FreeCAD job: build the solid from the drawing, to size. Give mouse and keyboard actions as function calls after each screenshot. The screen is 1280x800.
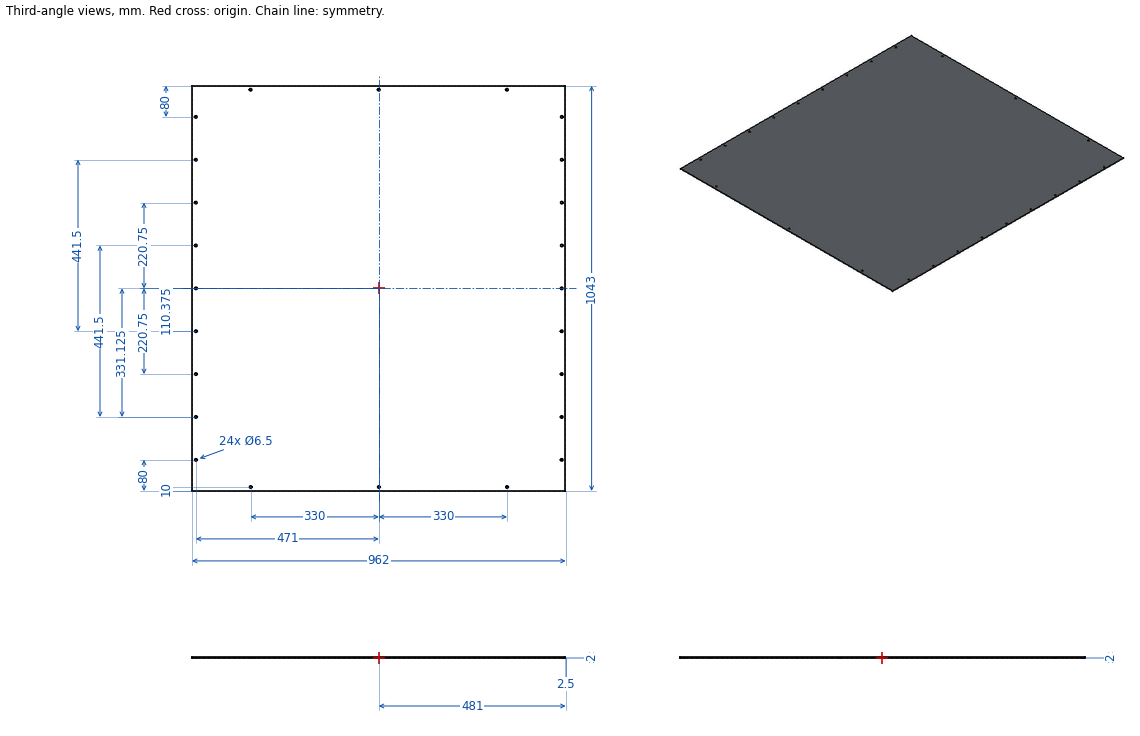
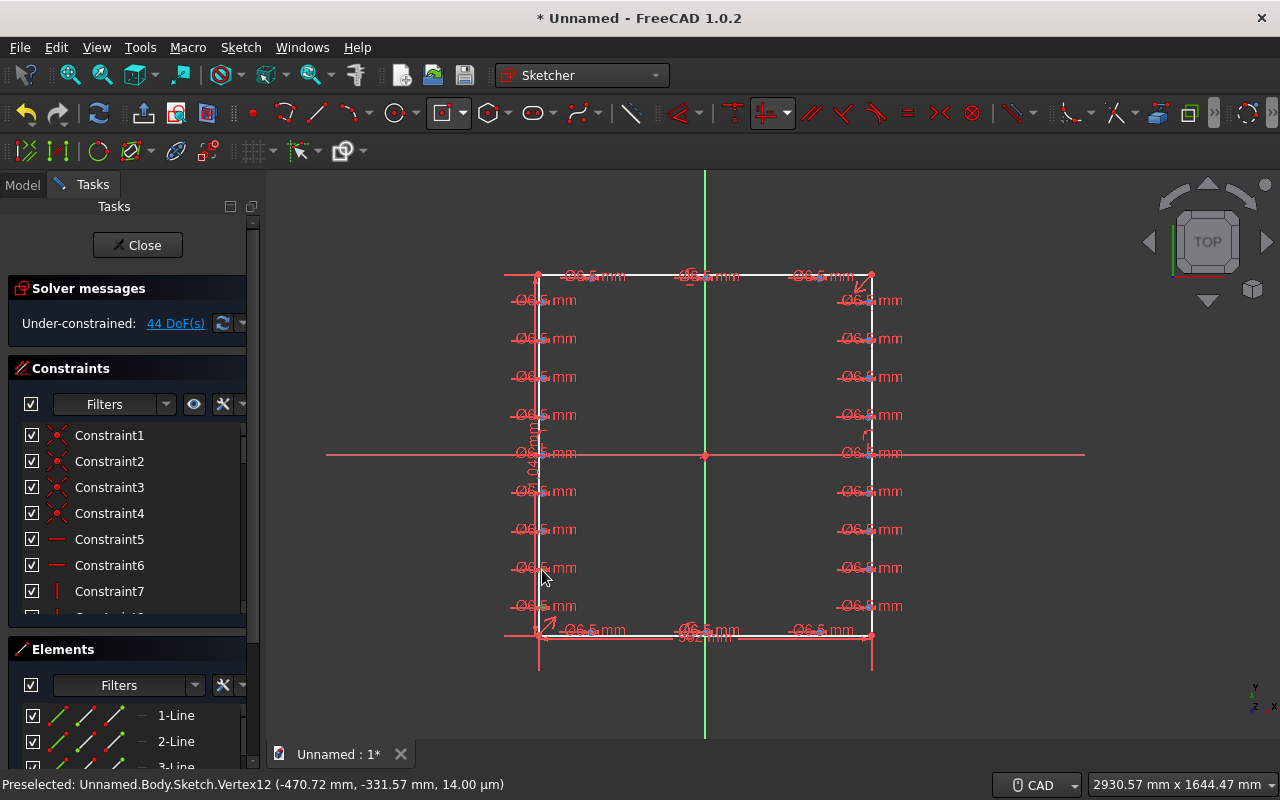
click(790, 114)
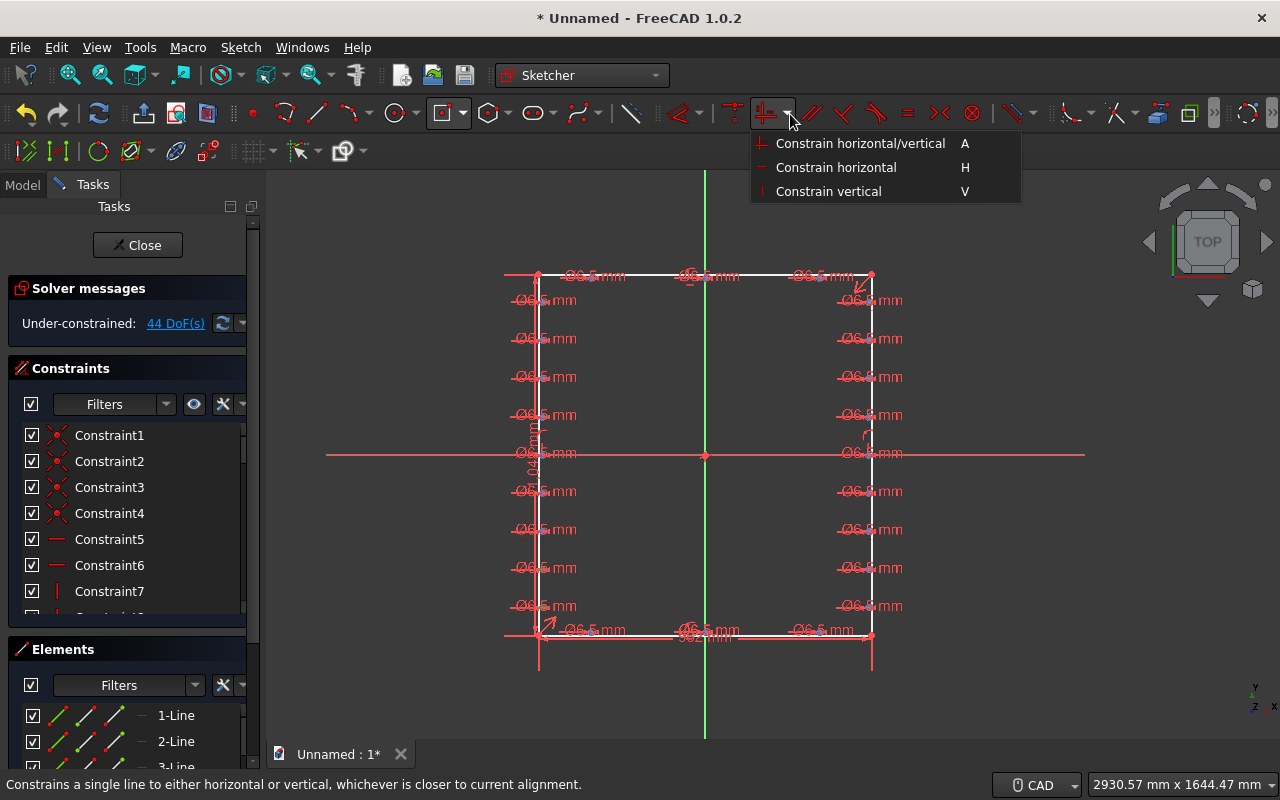
click(886, 191)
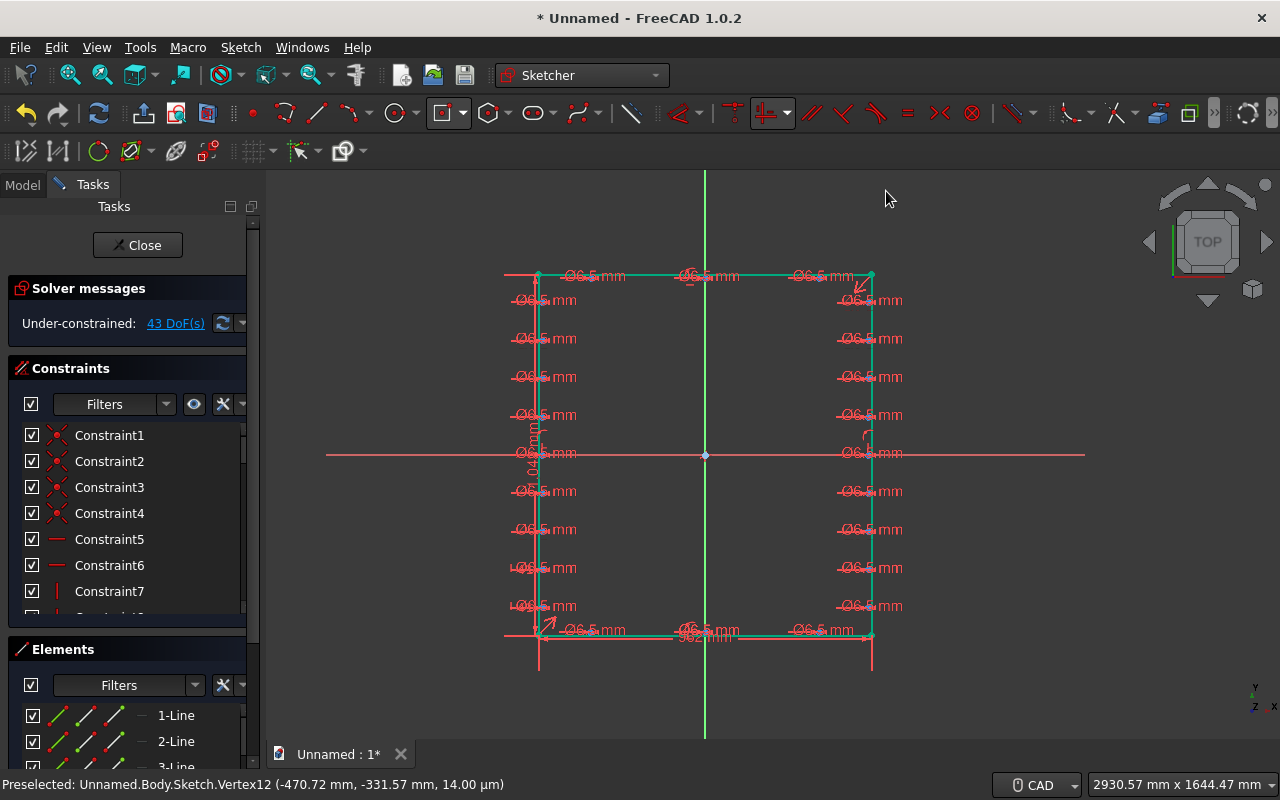
click(542, 570)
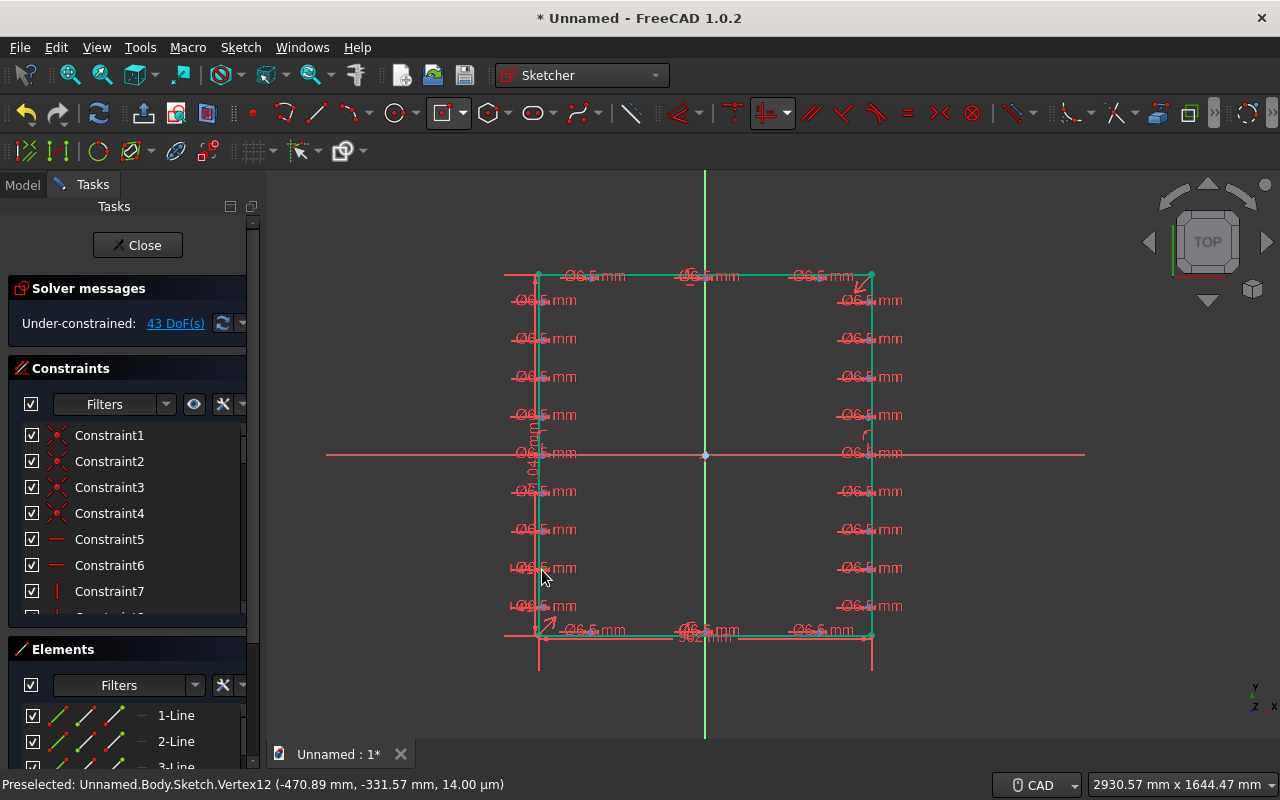
click(542, 532)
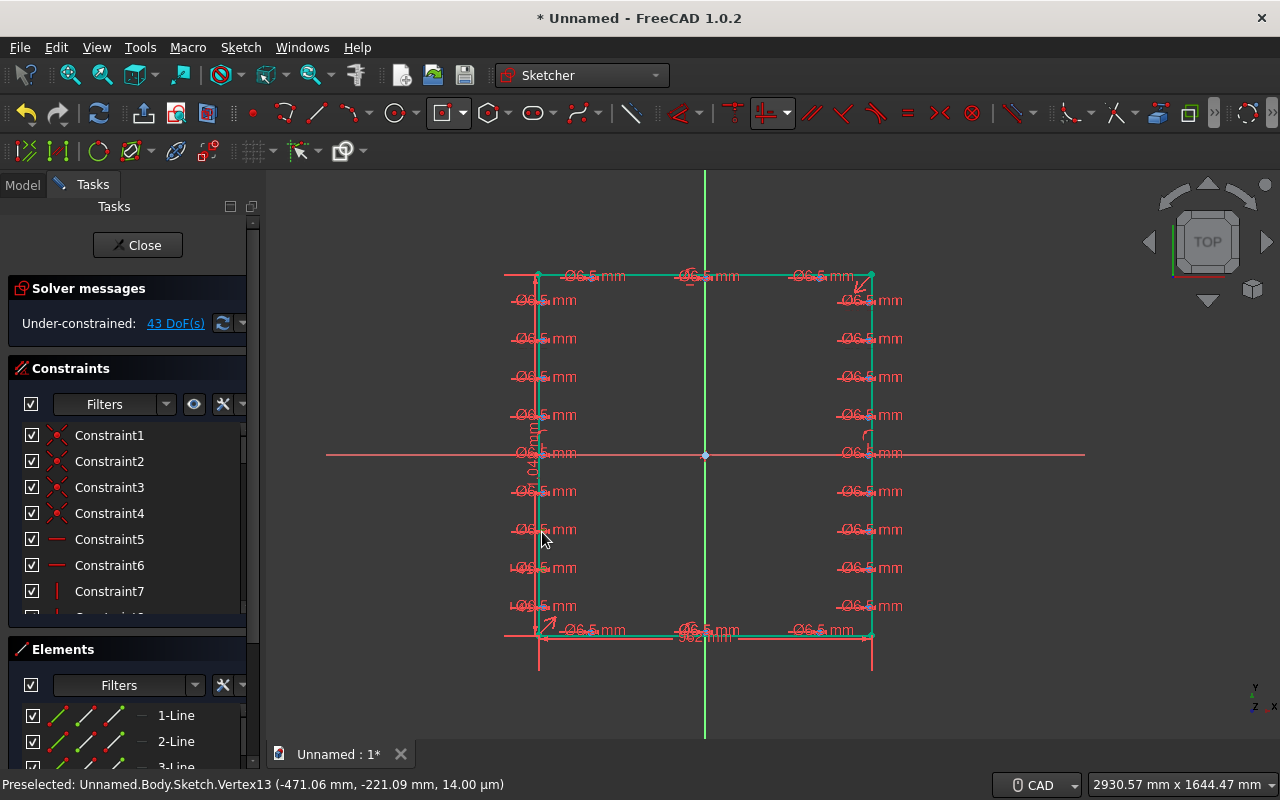
click(790, 114)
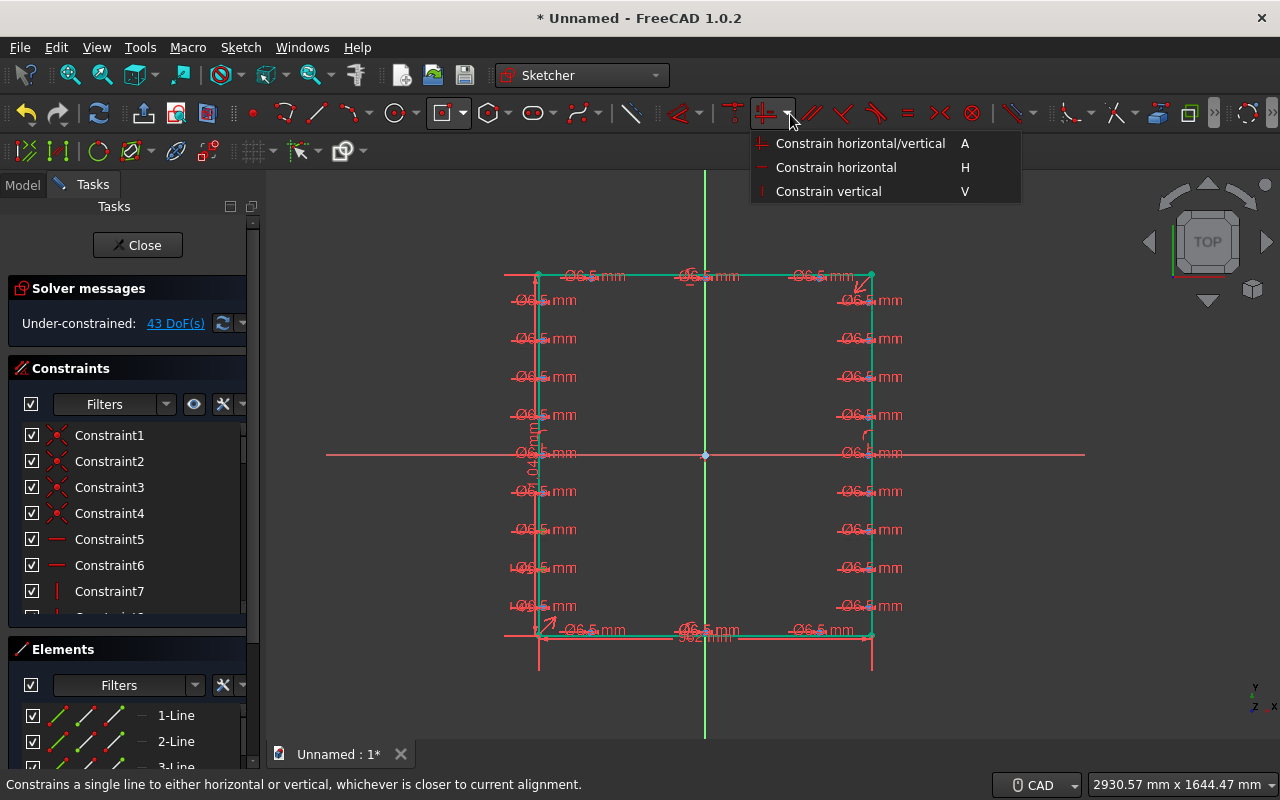
click(886, 191)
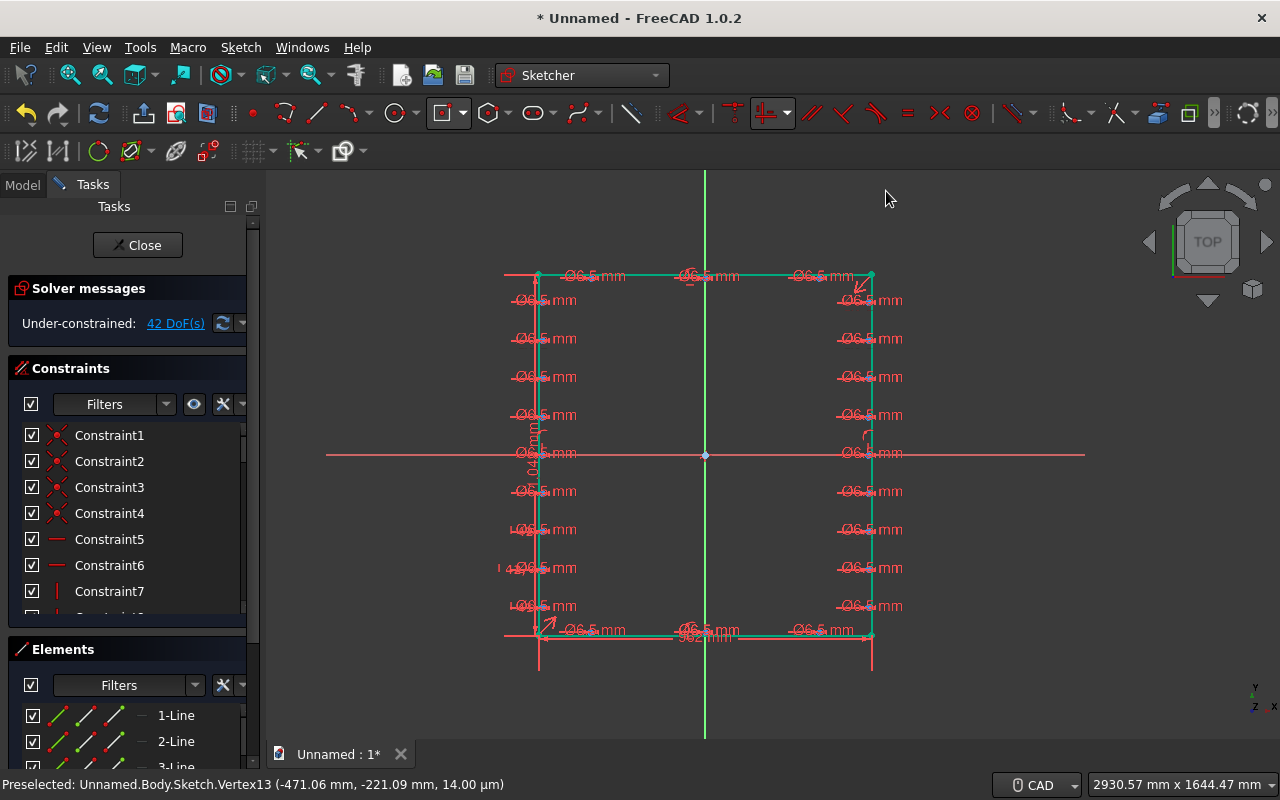
click(542, 532)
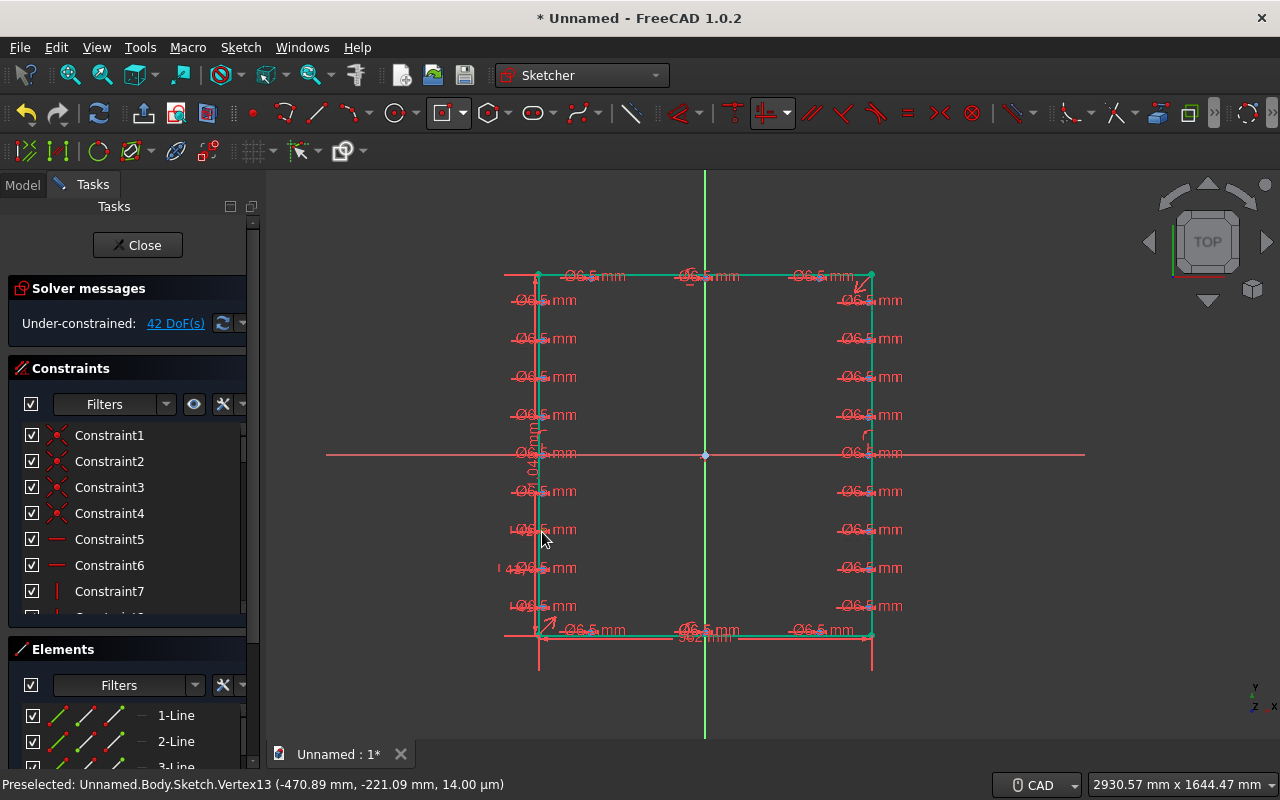
click(542, 493)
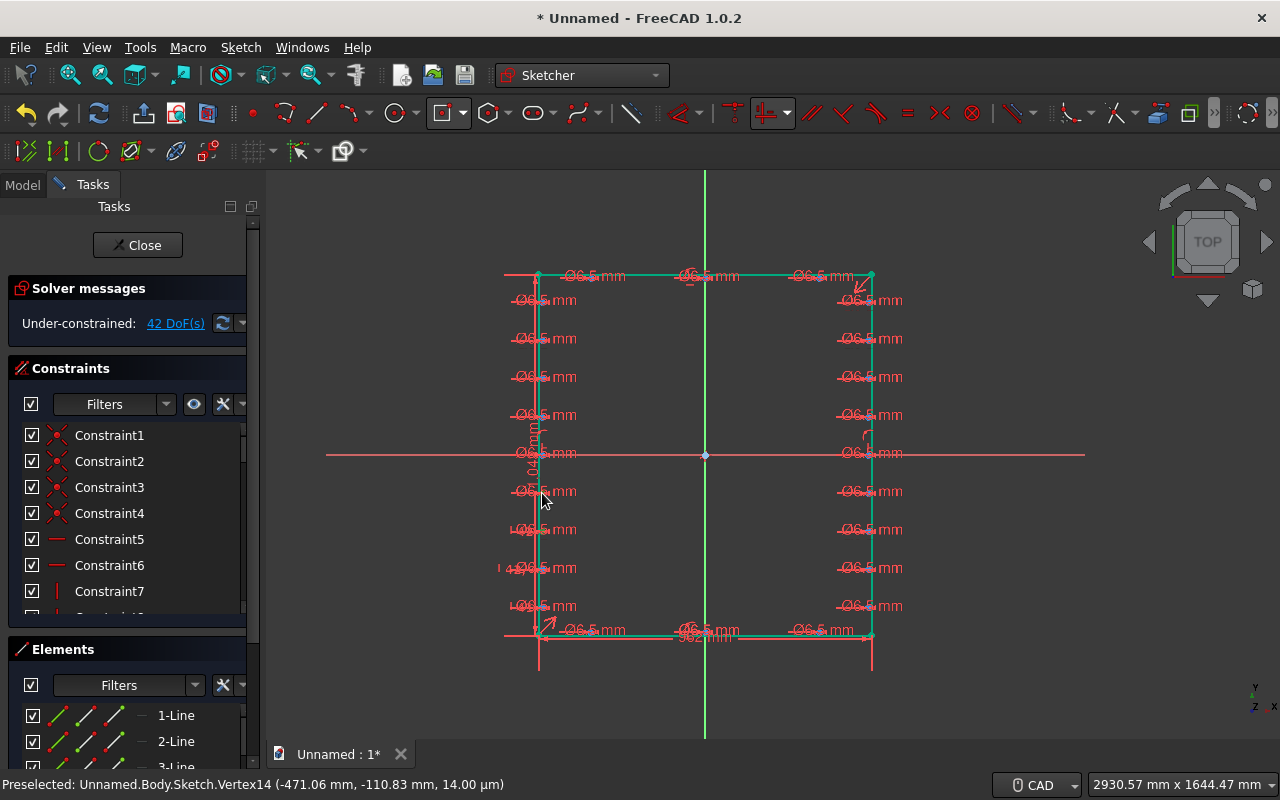
click(790, 114)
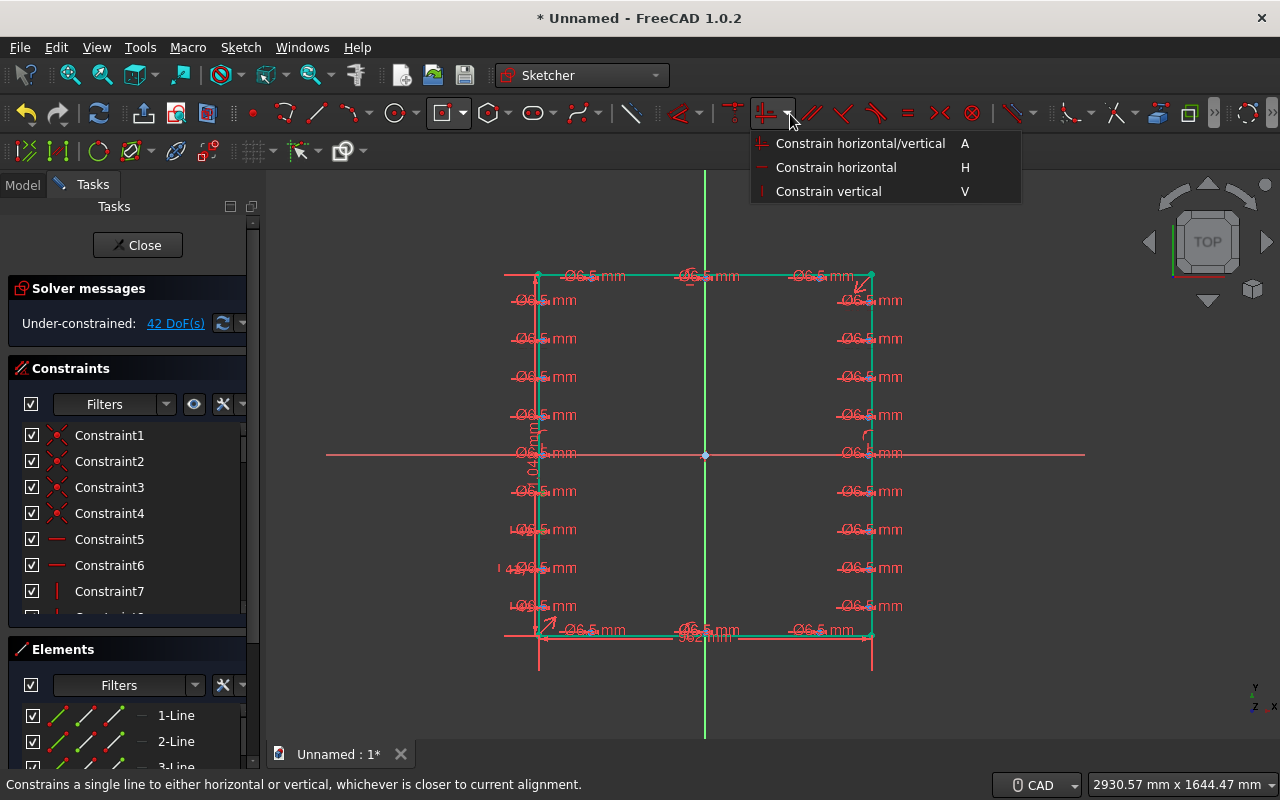
click(886, 191)